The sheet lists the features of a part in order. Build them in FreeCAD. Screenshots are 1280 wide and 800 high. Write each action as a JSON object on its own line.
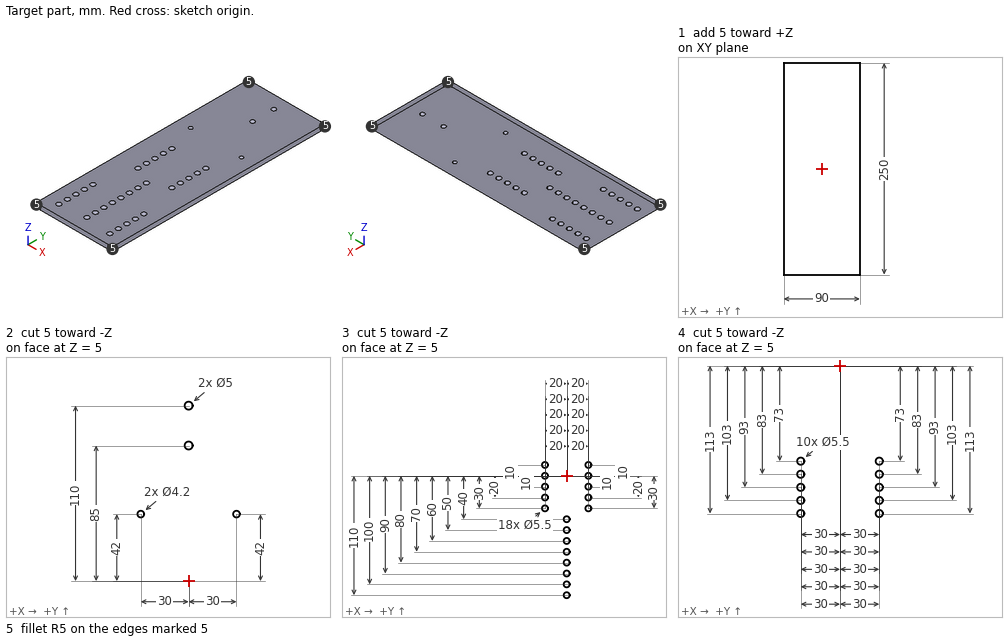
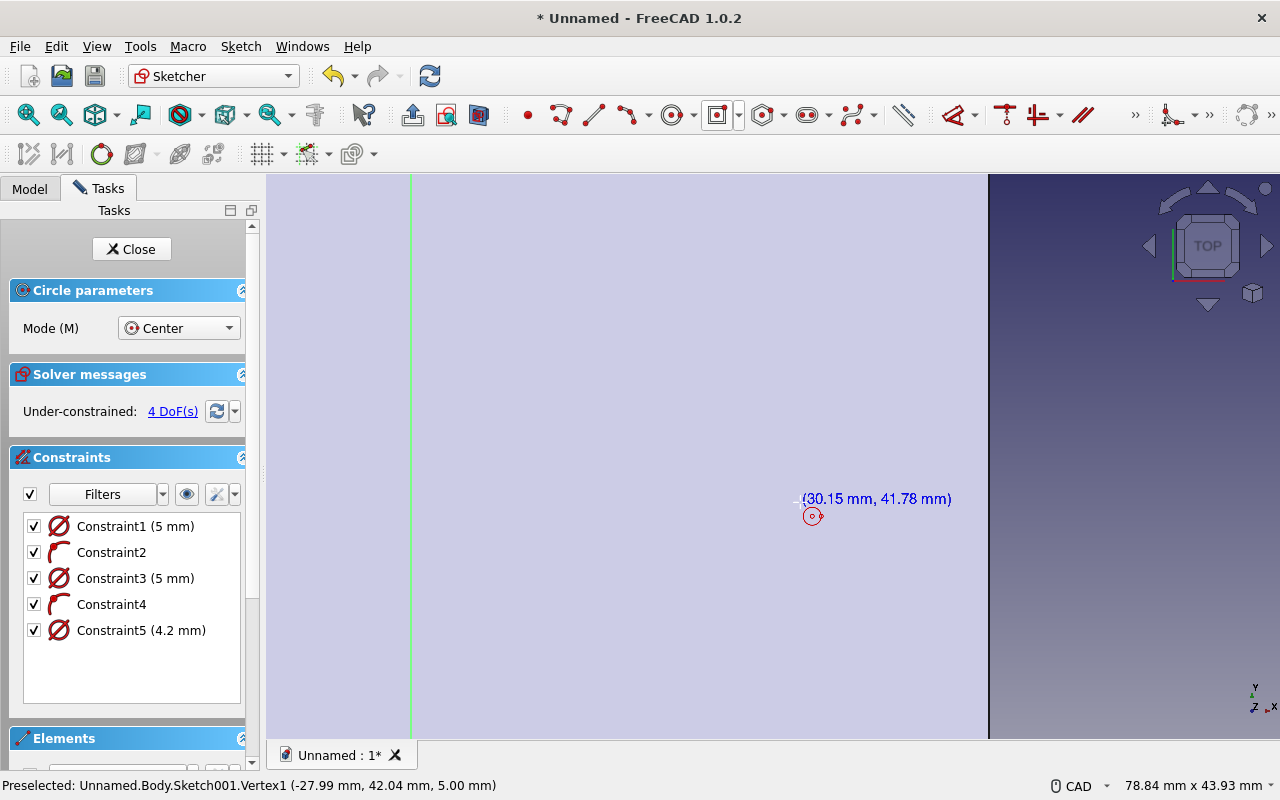
{"action": "scroll", "coordinate": [801, 502], "scroll_direction": "down", "scroll_amount": 7}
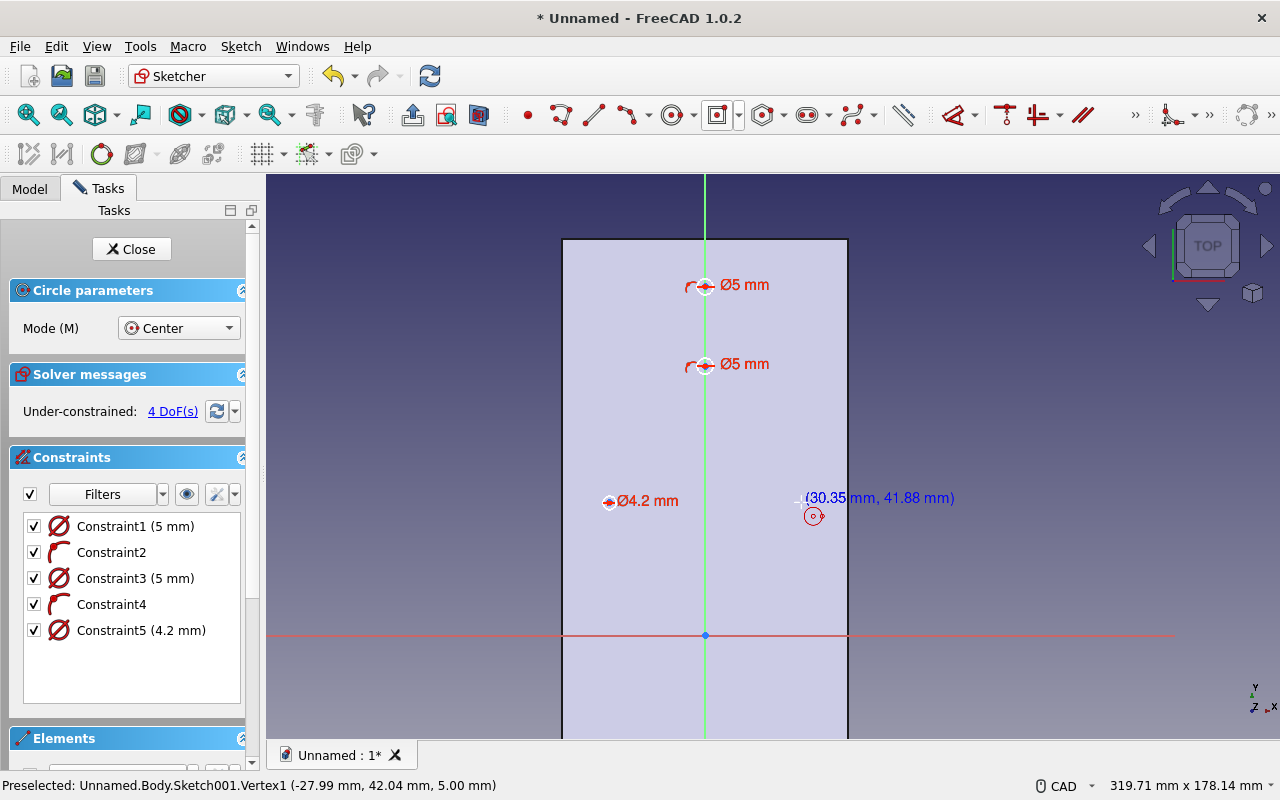
{"action": "left_click", "coordinate": [800, 502]}
{"action": "mouse_move", "coordinate": [805, 498]}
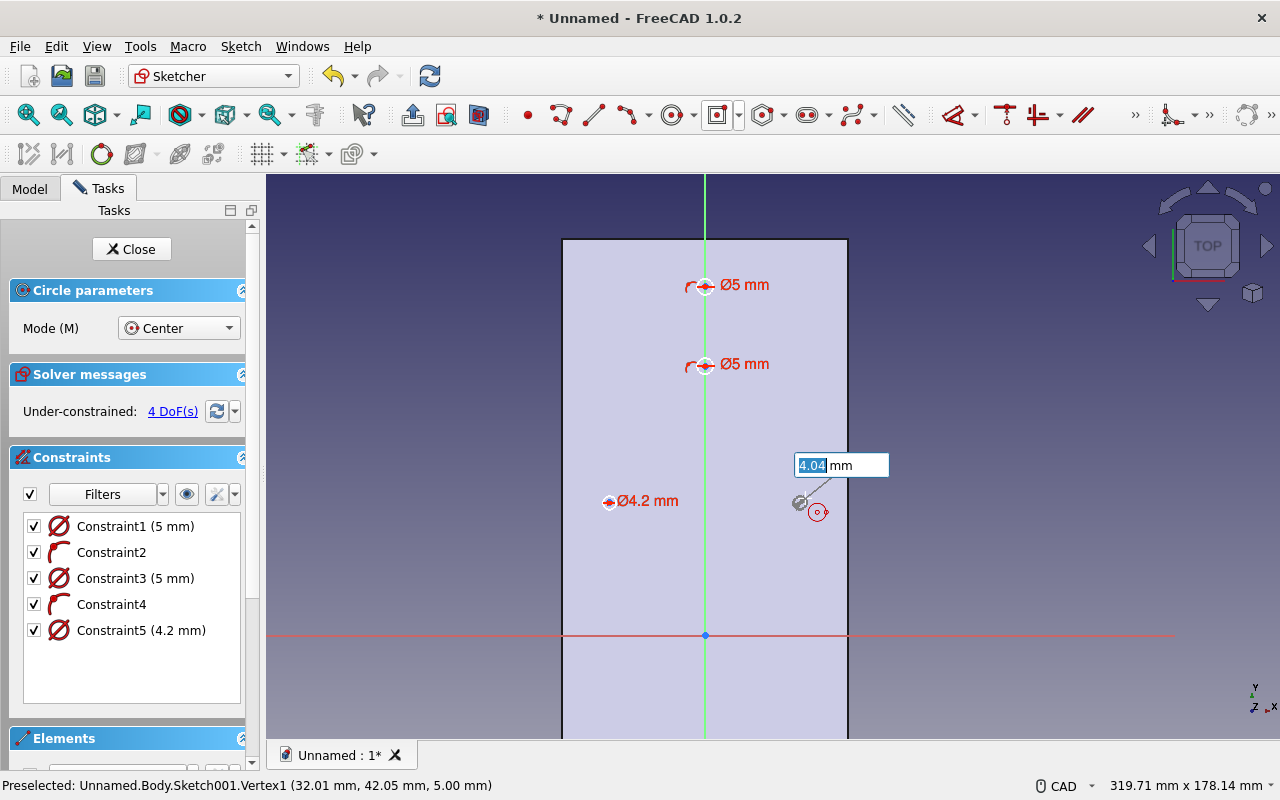
{"action": "type", "text": "4.2"}
{"action": "key", "text": "Return"}
{"action": "key", "text": "Escape"}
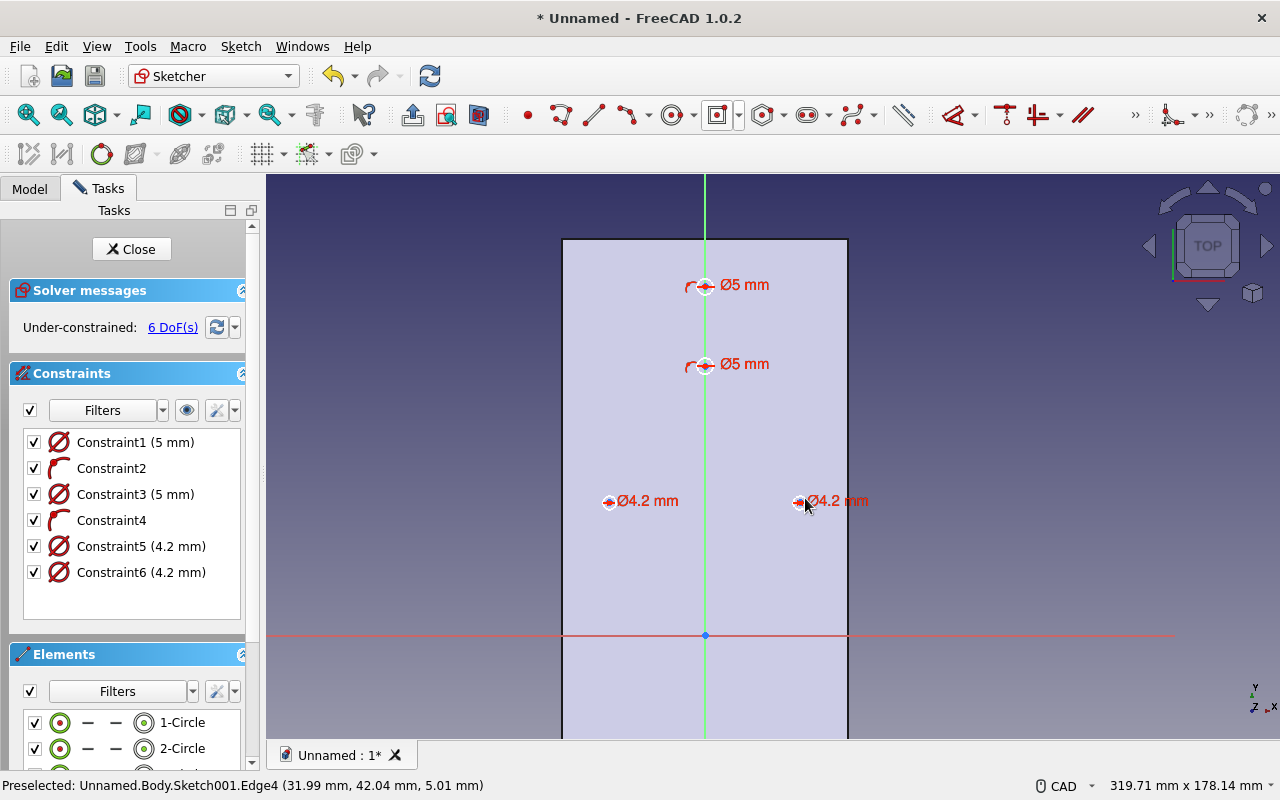
{"action": "key", "text": "d"}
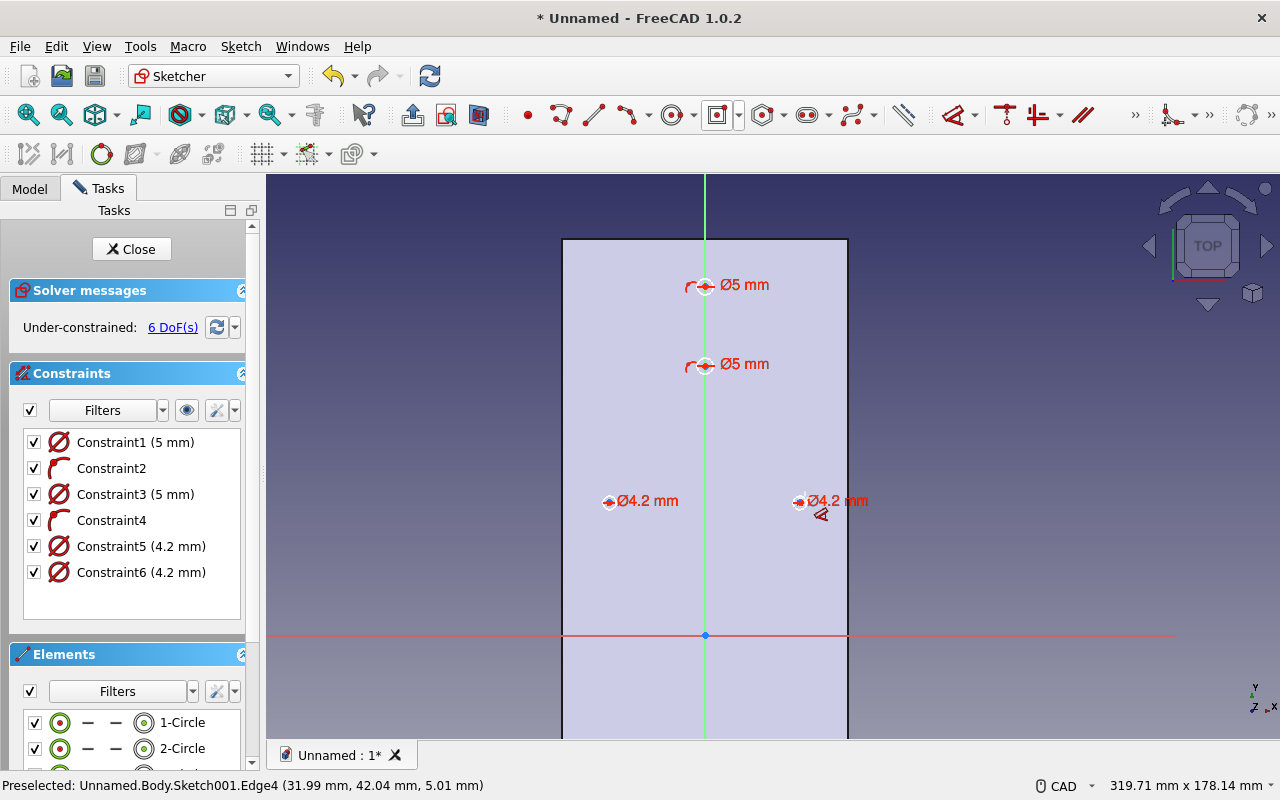
{"action": "left_click", "coordinate": [705, 366]}
{"action": "left_click", "coordinate": [739, 501]}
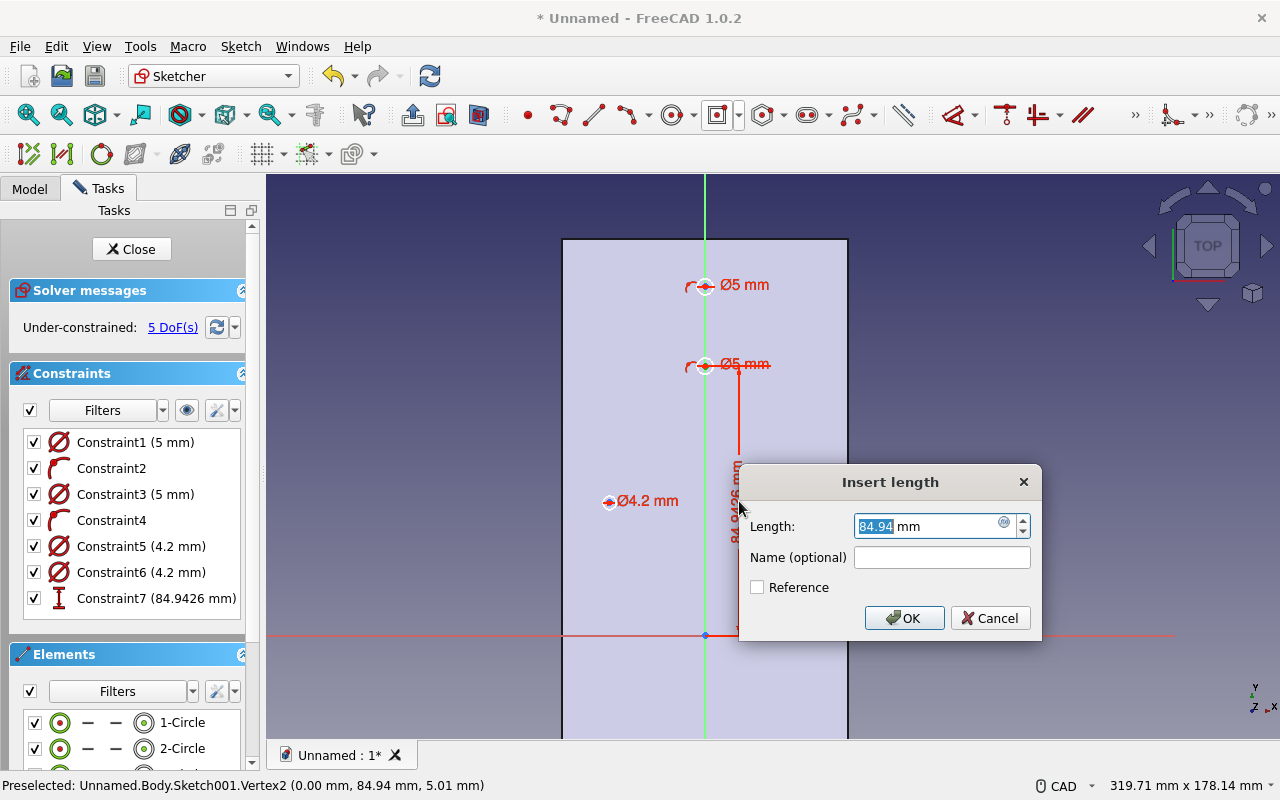
{"action": "type", "text": "85"}
{"action": "key", "text": "Return"}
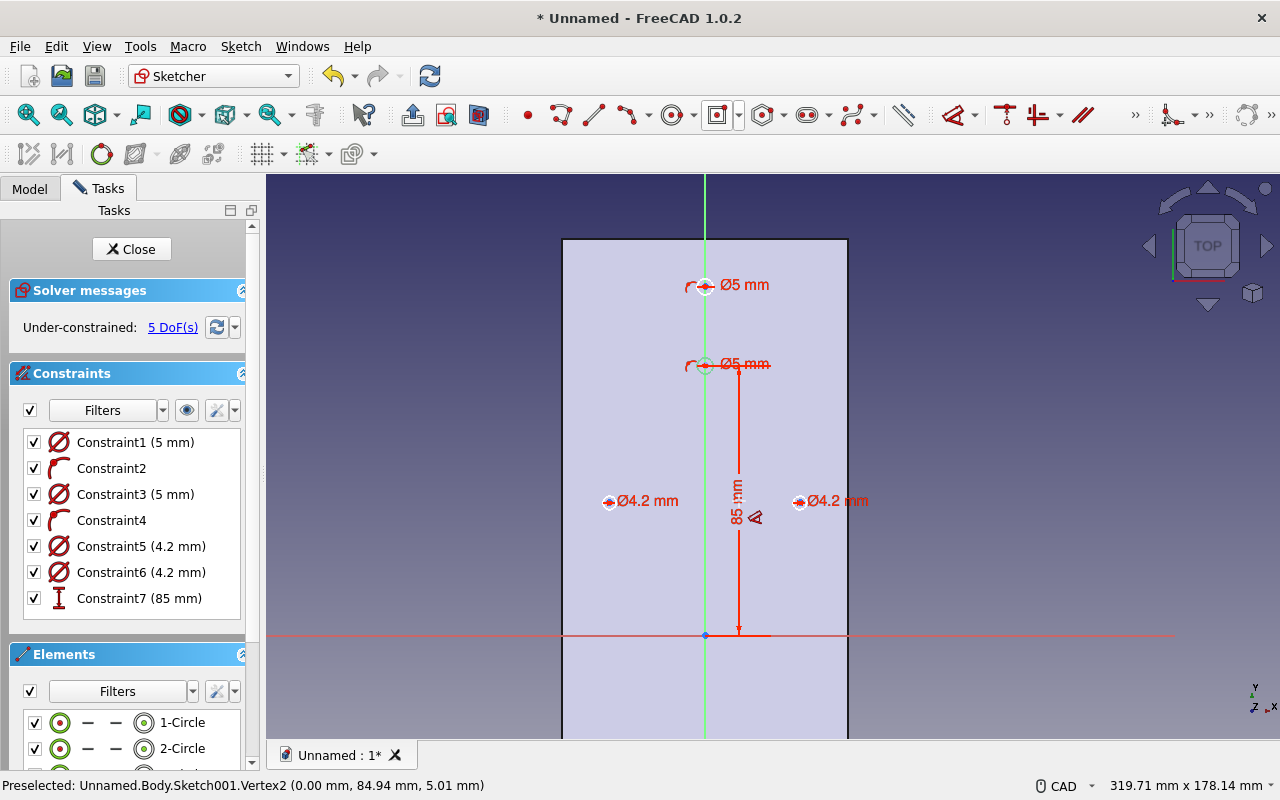
{"action": "left_click", "coordinate": [610, 503]}
{"action": "left_click", "coordinate": [657, 670]}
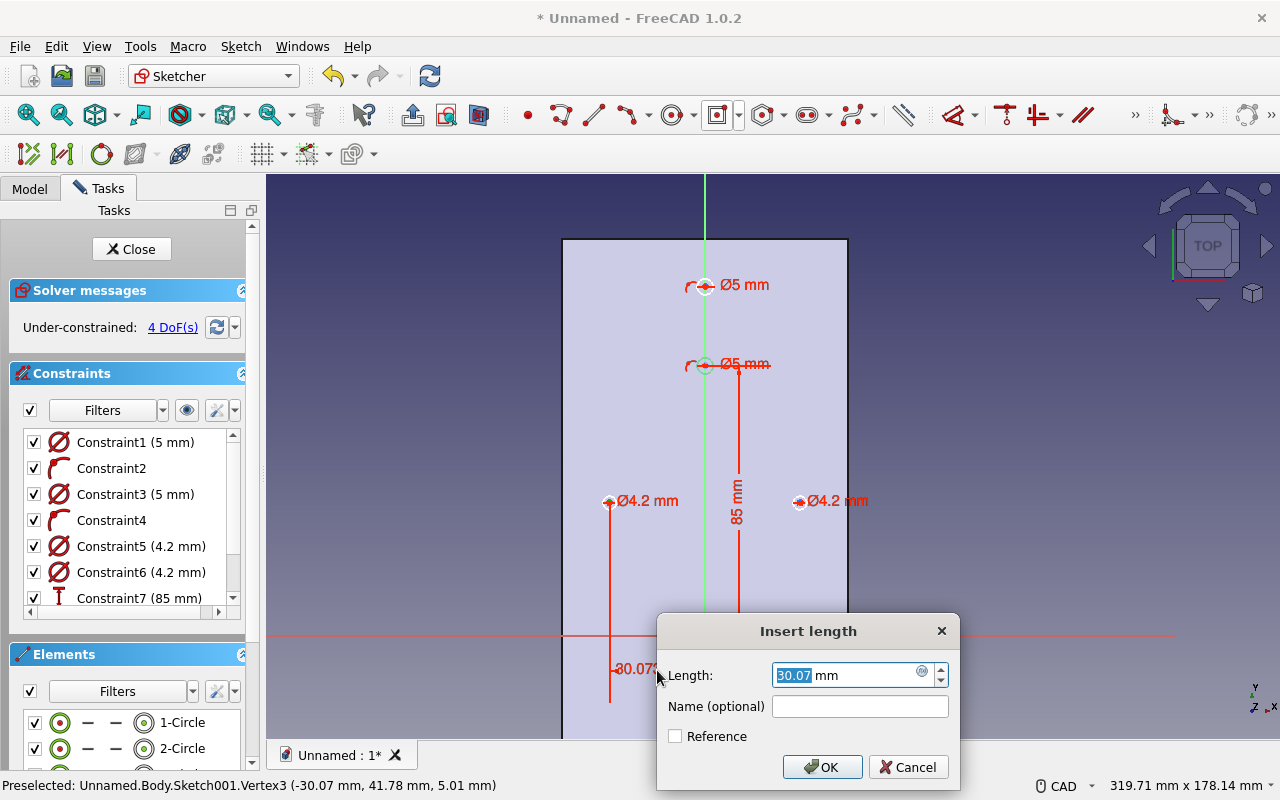
{"action": "type", "text": "30"}
{"action": "key", "text": "Return"}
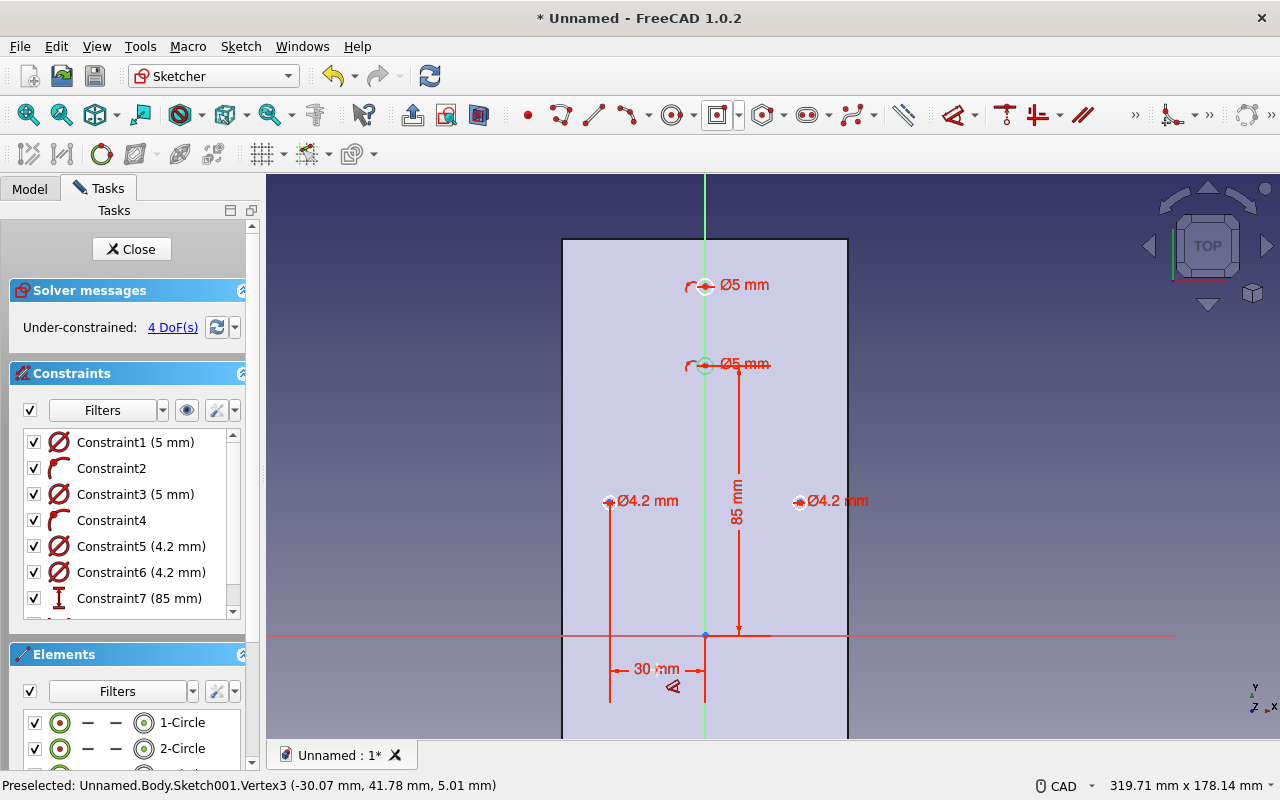
{"action": "left_click", "coordinate": [610, 503]}
{"action": "left_click", "coordinate": [576, 569]}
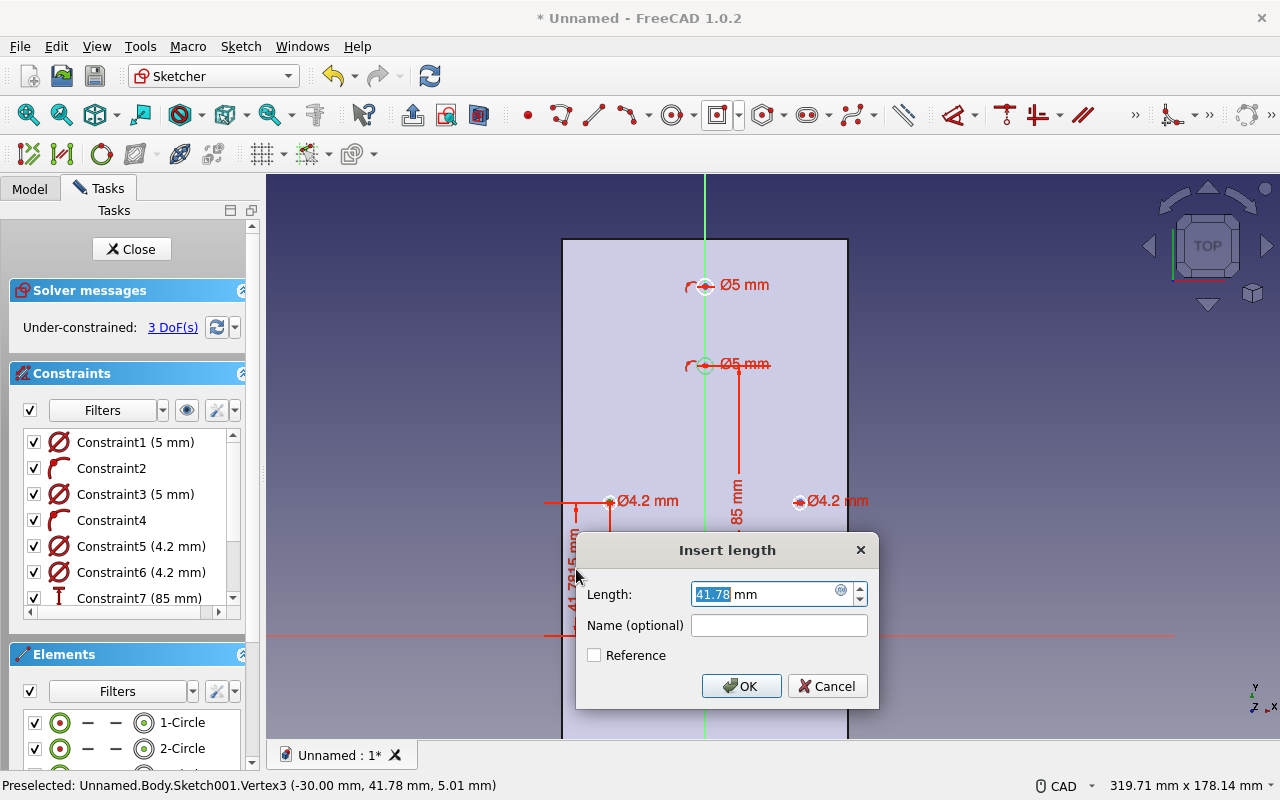
{"action": "type", "text": "42"}
{"action": "key", "text": "Return"}